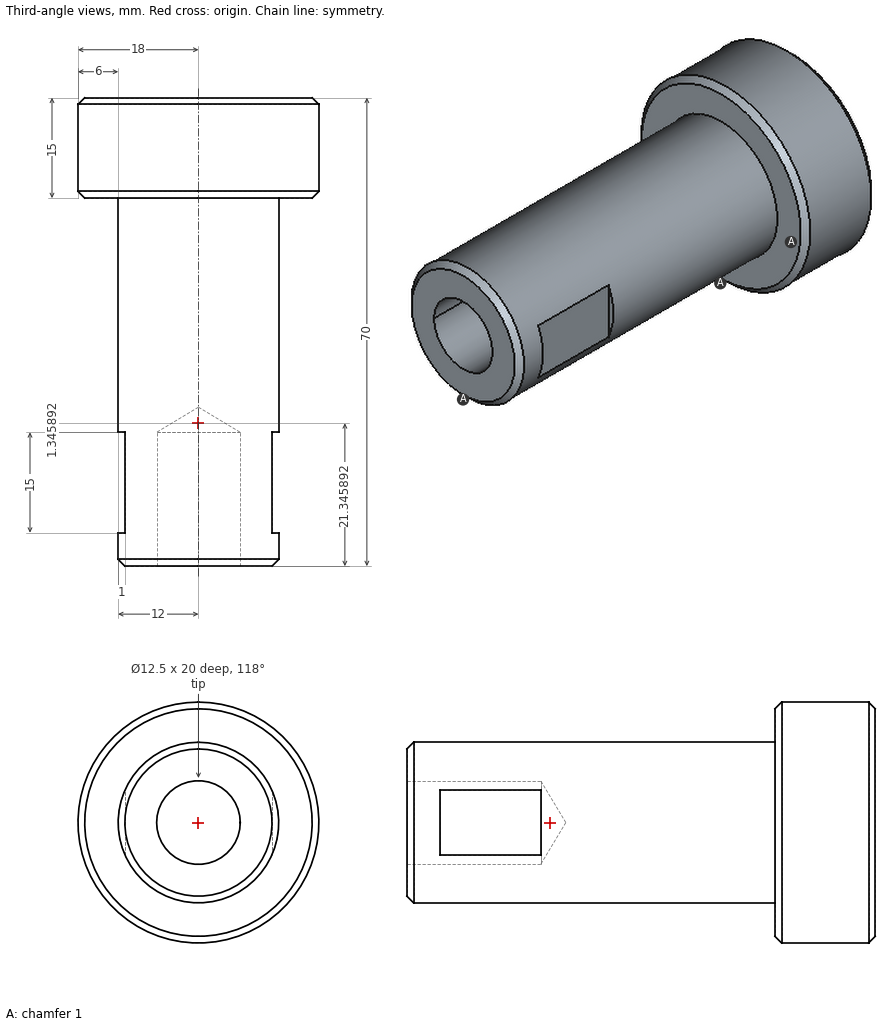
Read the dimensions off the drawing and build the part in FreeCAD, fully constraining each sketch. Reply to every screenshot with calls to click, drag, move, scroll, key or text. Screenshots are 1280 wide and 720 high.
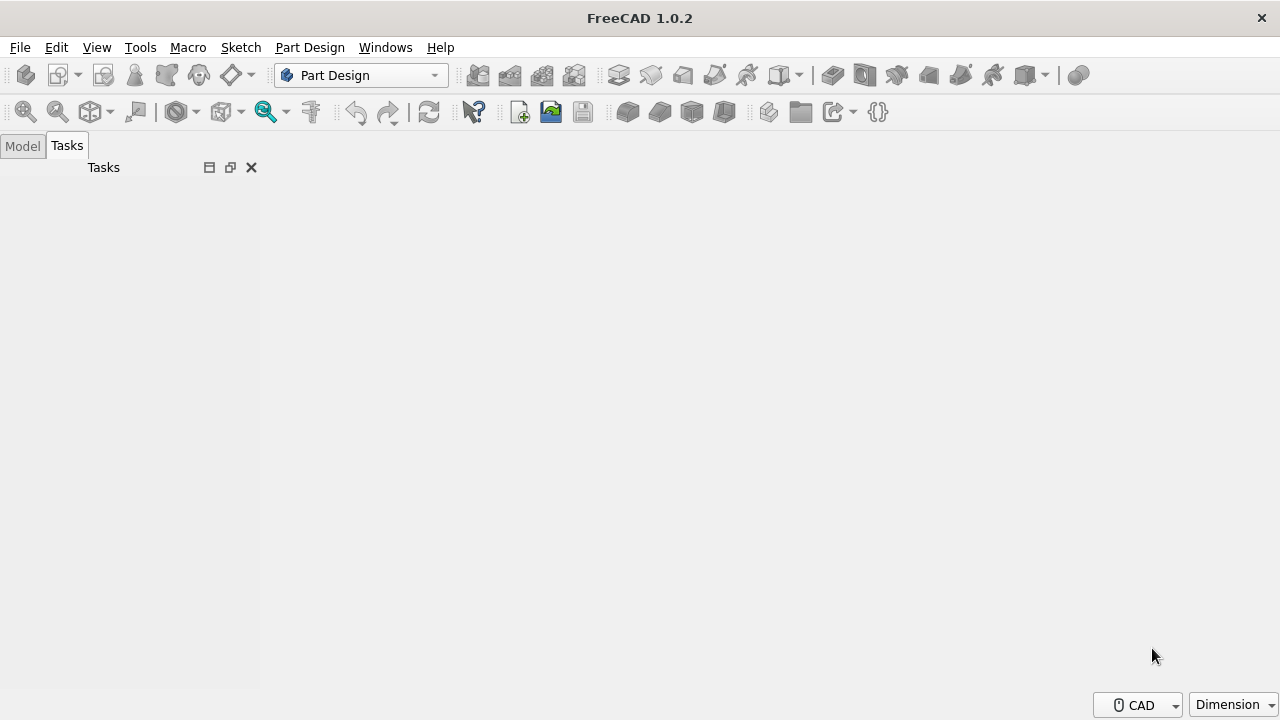
click(520, 112)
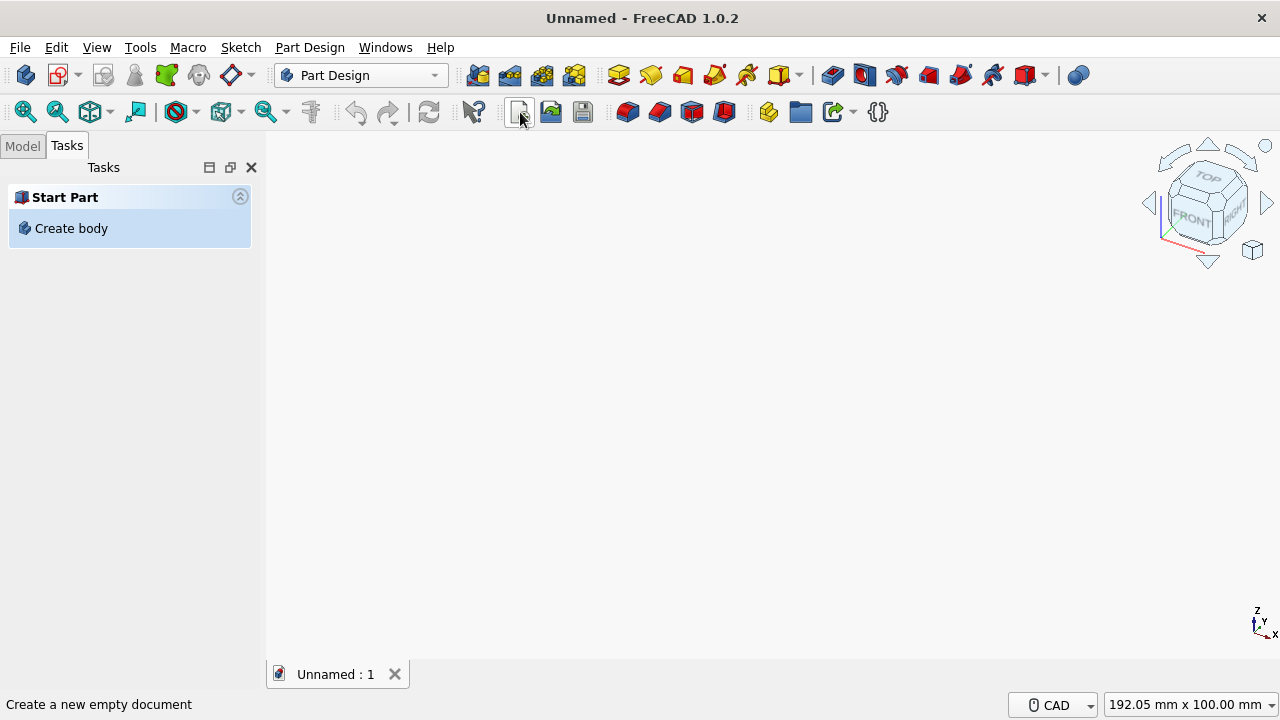
click(58, 76)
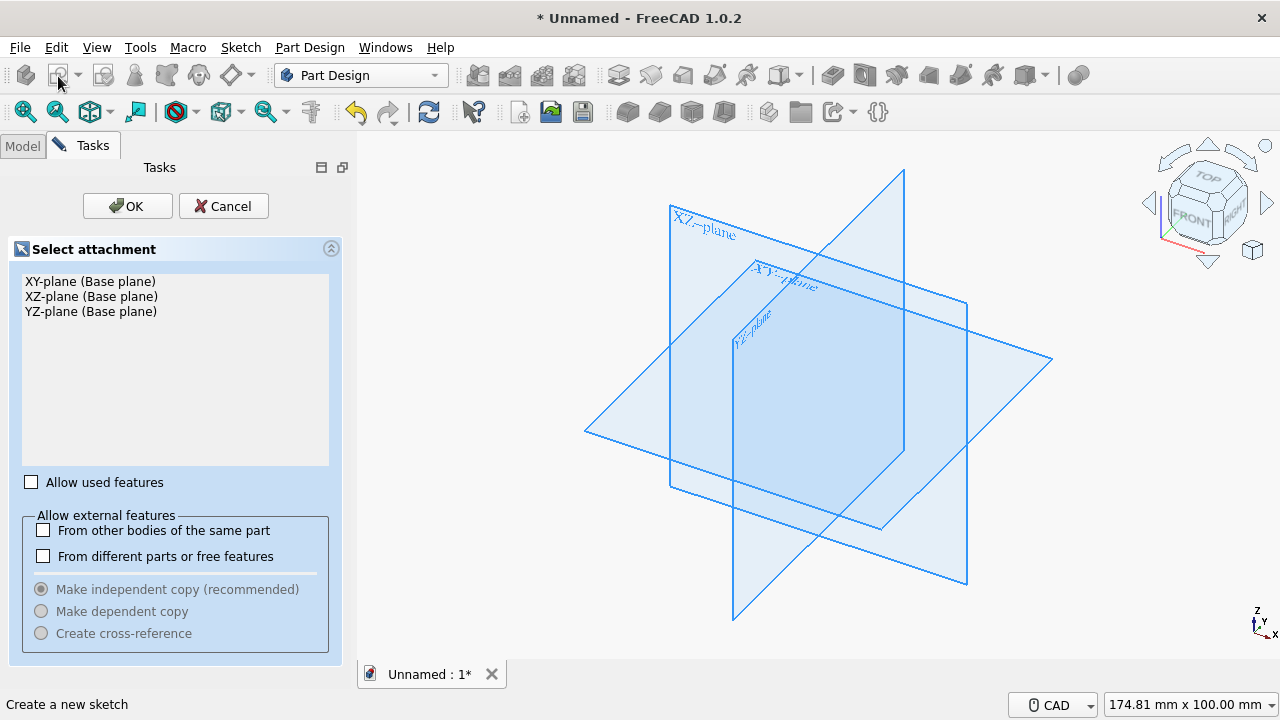
click(82, 282)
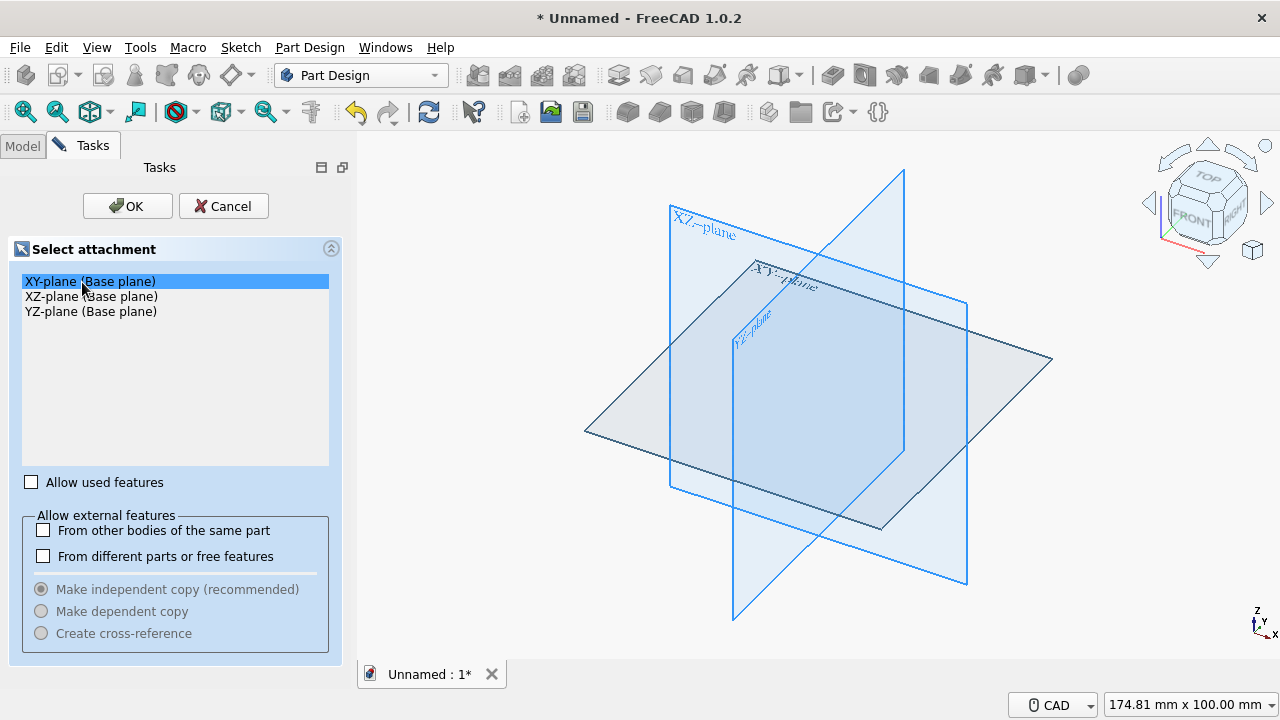
click(128, 206)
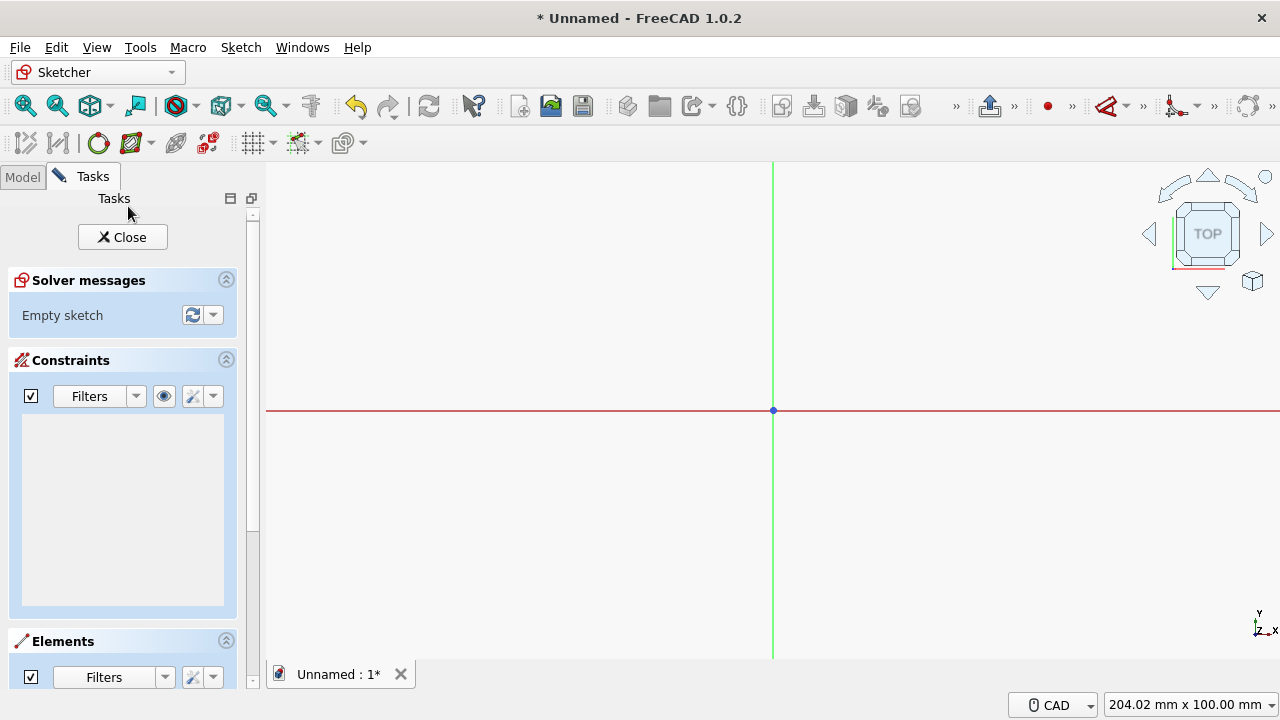
scroll(597, 631, down, 1)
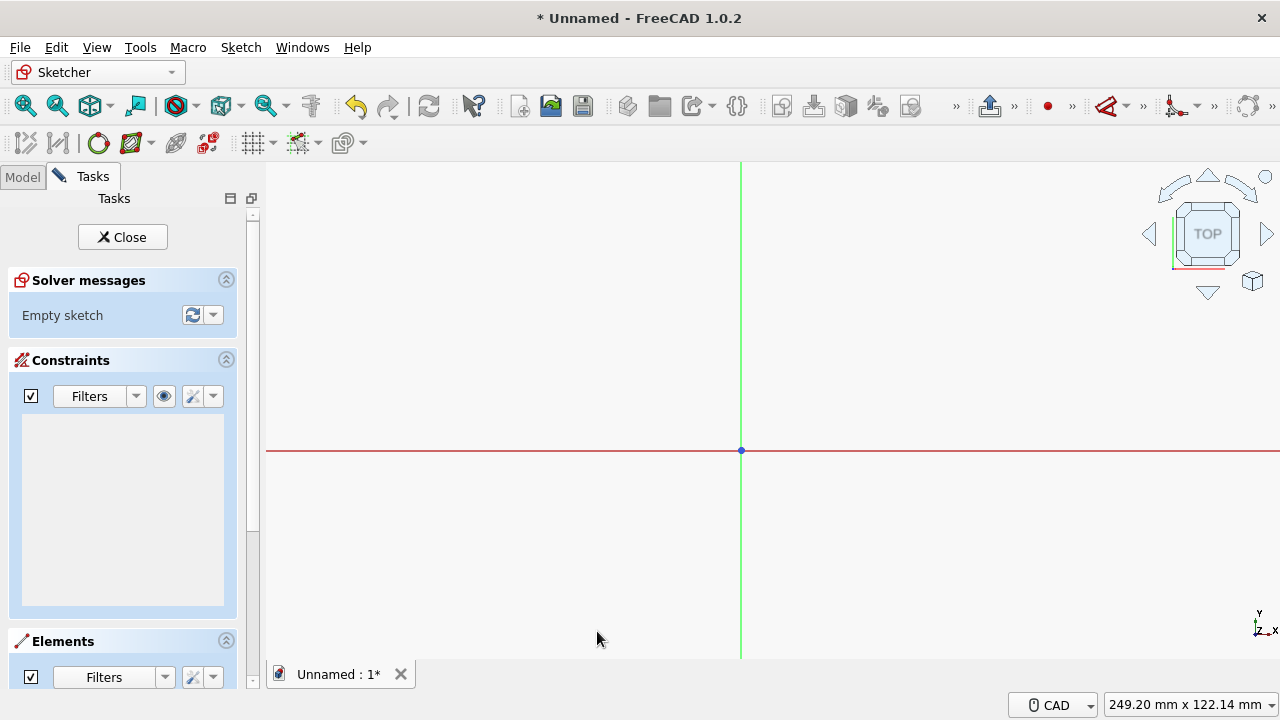
key(g)
key(m)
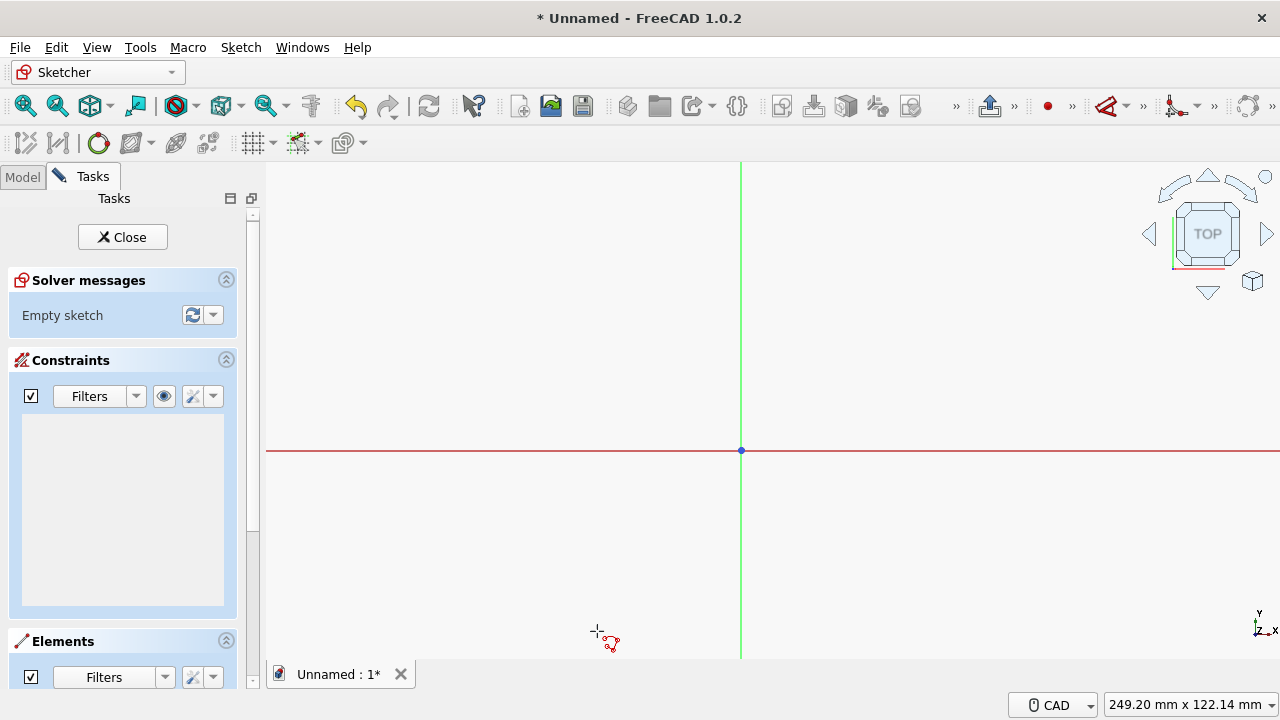
click(741, 537)
click(732, 253)
click(668, 253)
click(668, 314)
click(692, 314)
click(692, 537)
click(741, 538)
key(Escape)
key(Escape)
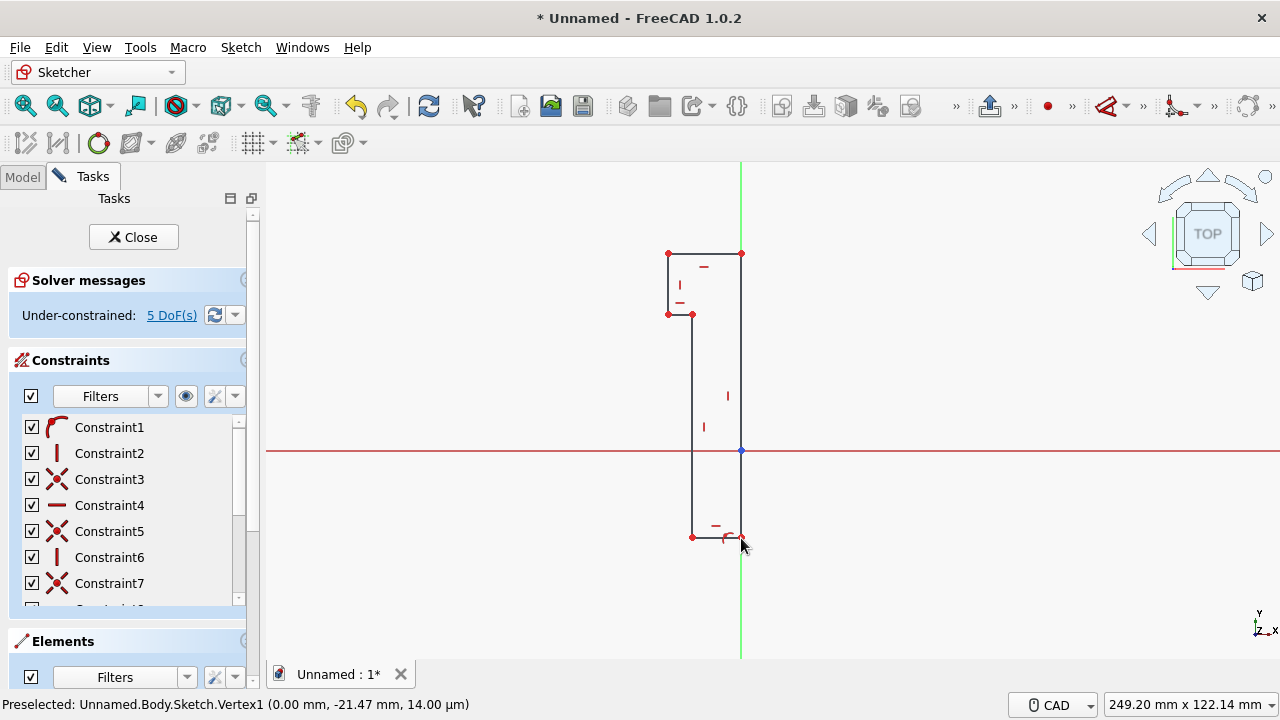
click(1106, 106)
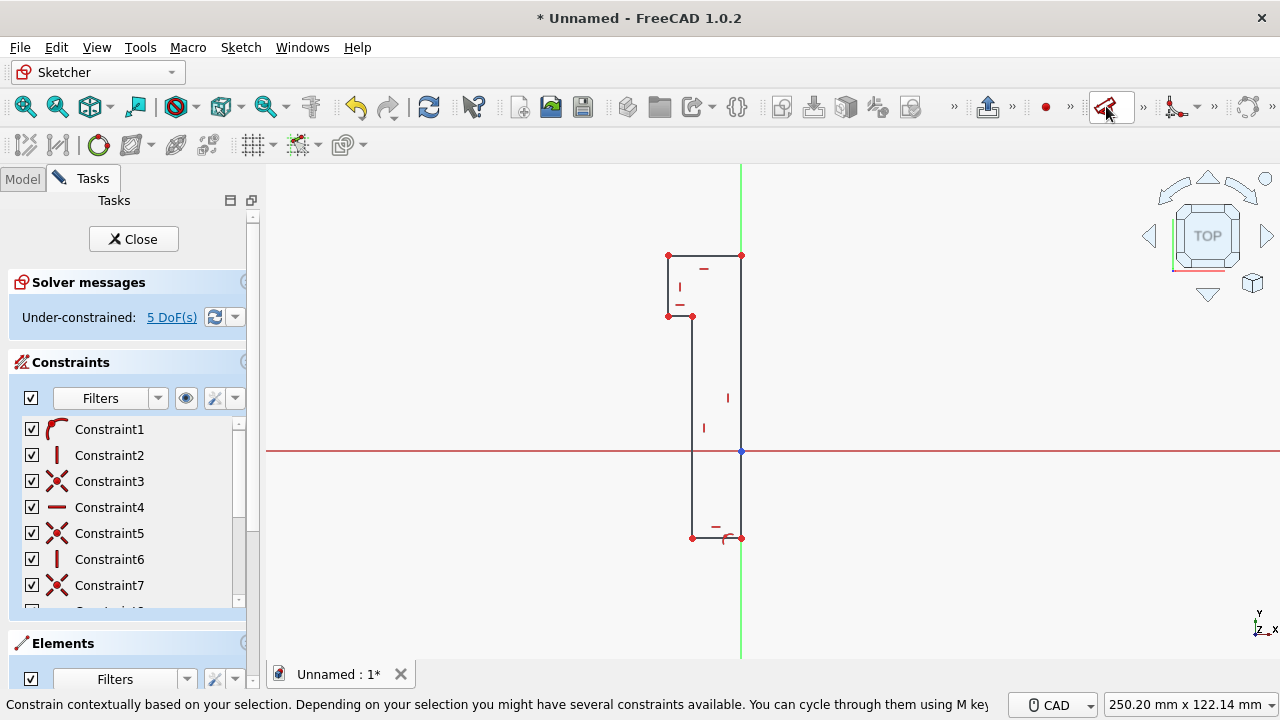
scroll(678, 316, up, 3)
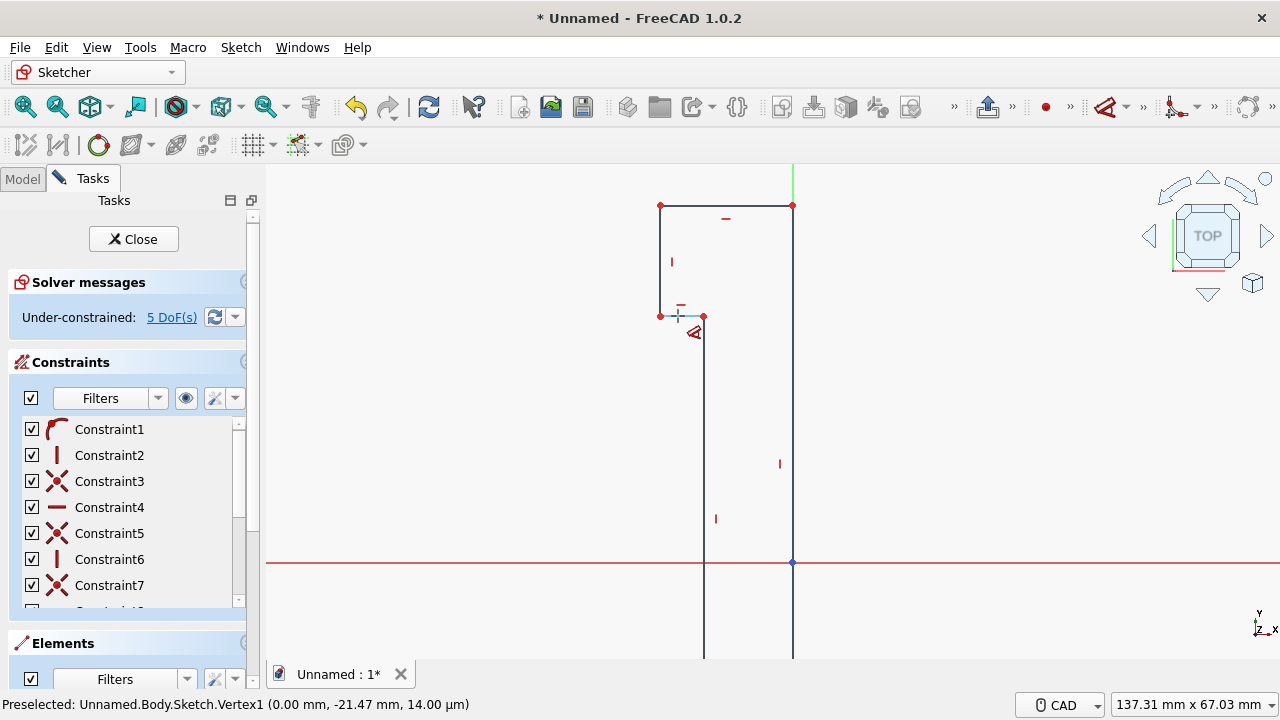
click(678, 316)
click(682, 282)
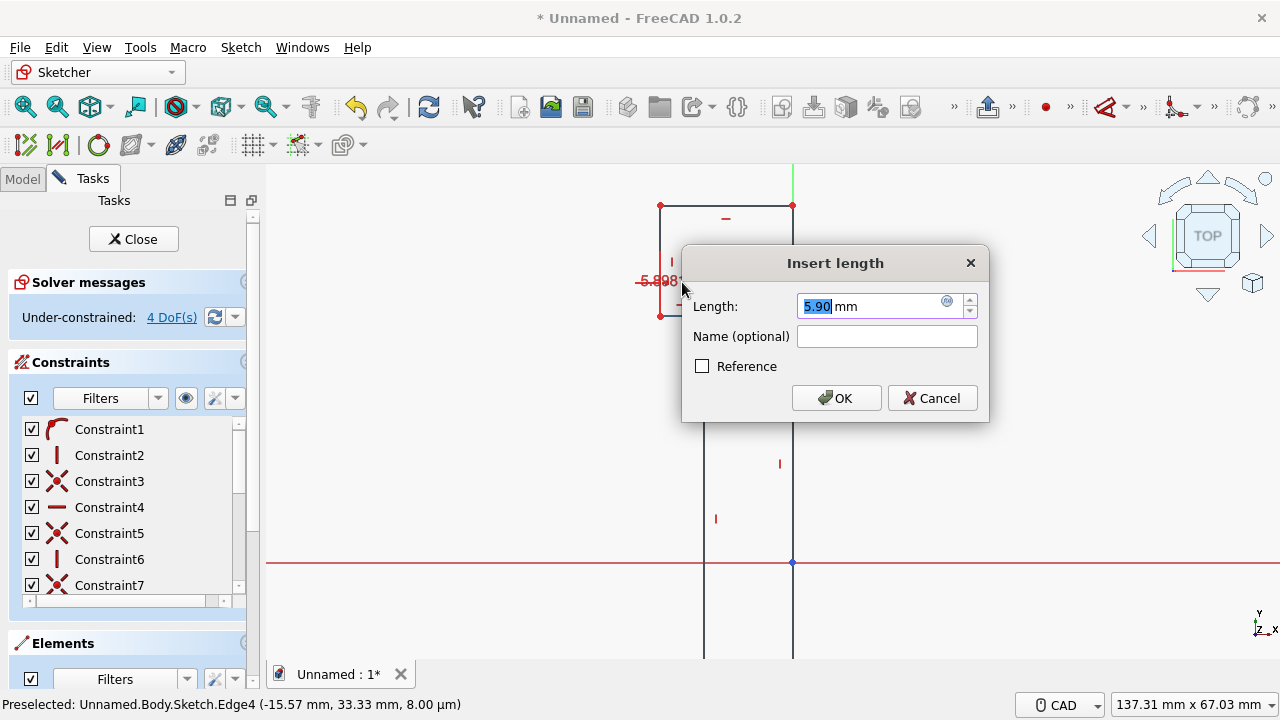
text(6)
key(Return)